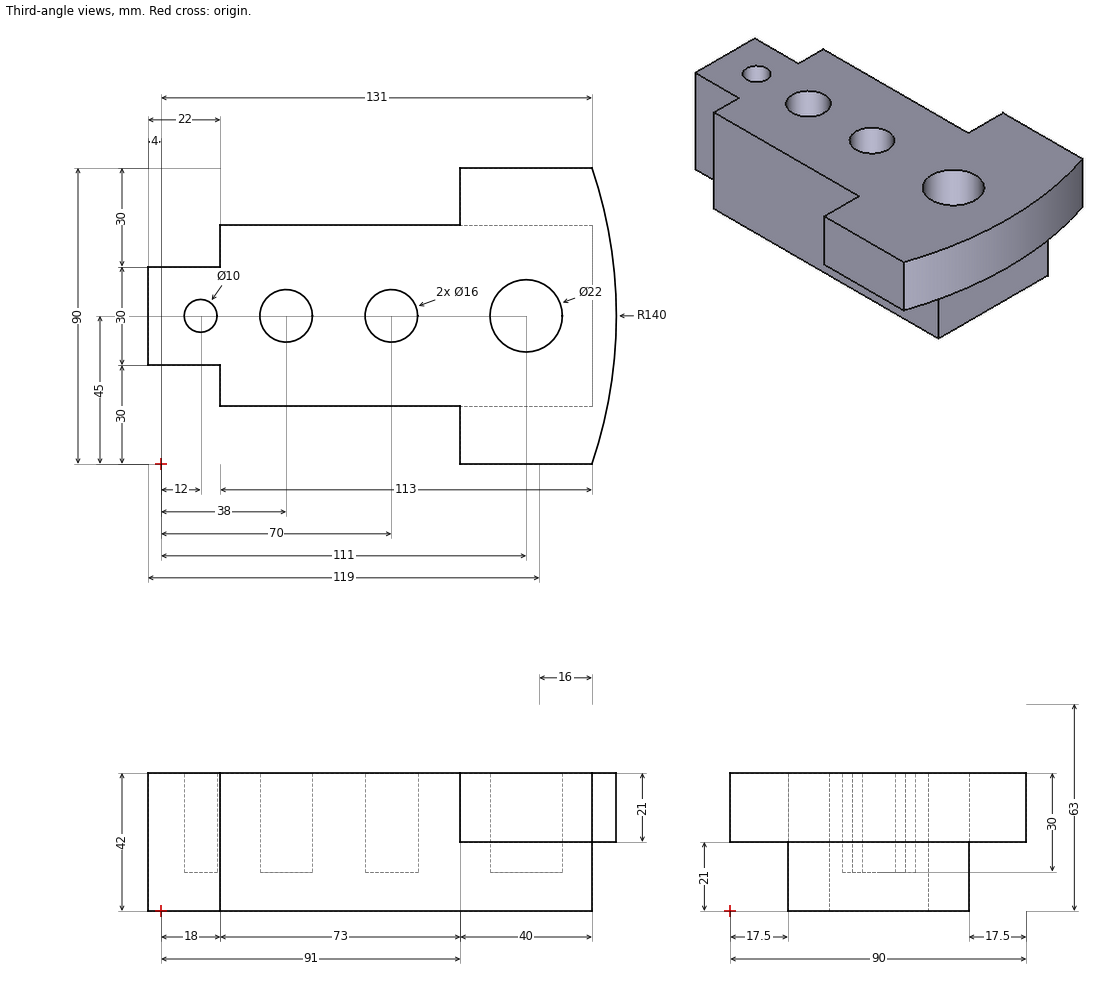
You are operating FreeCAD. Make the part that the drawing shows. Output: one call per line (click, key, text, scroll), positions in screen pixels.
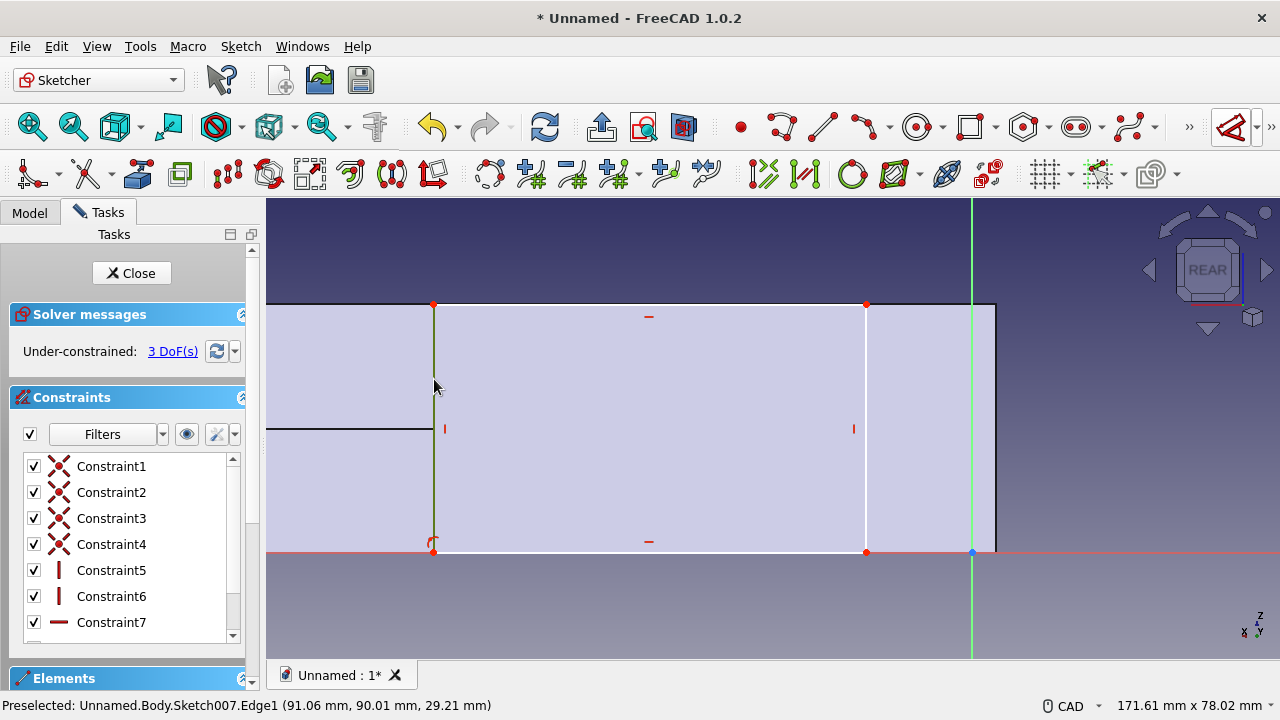
key(i)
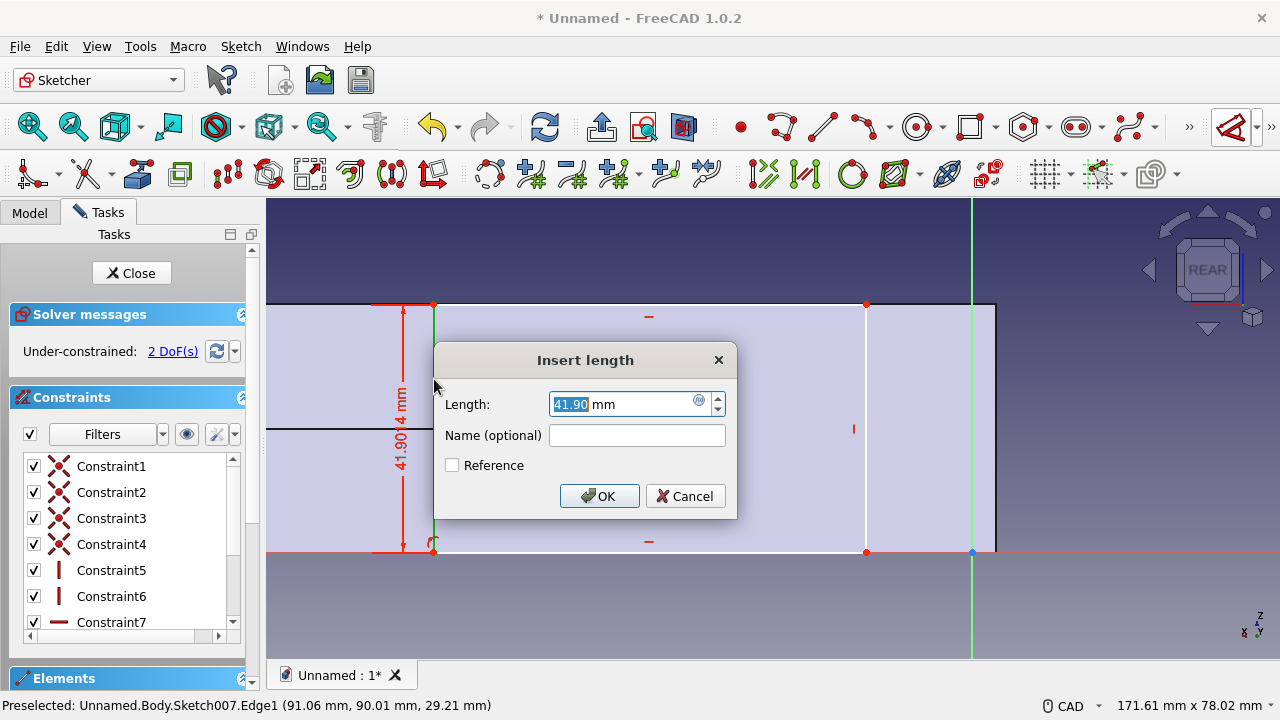
text(42)
key(Return)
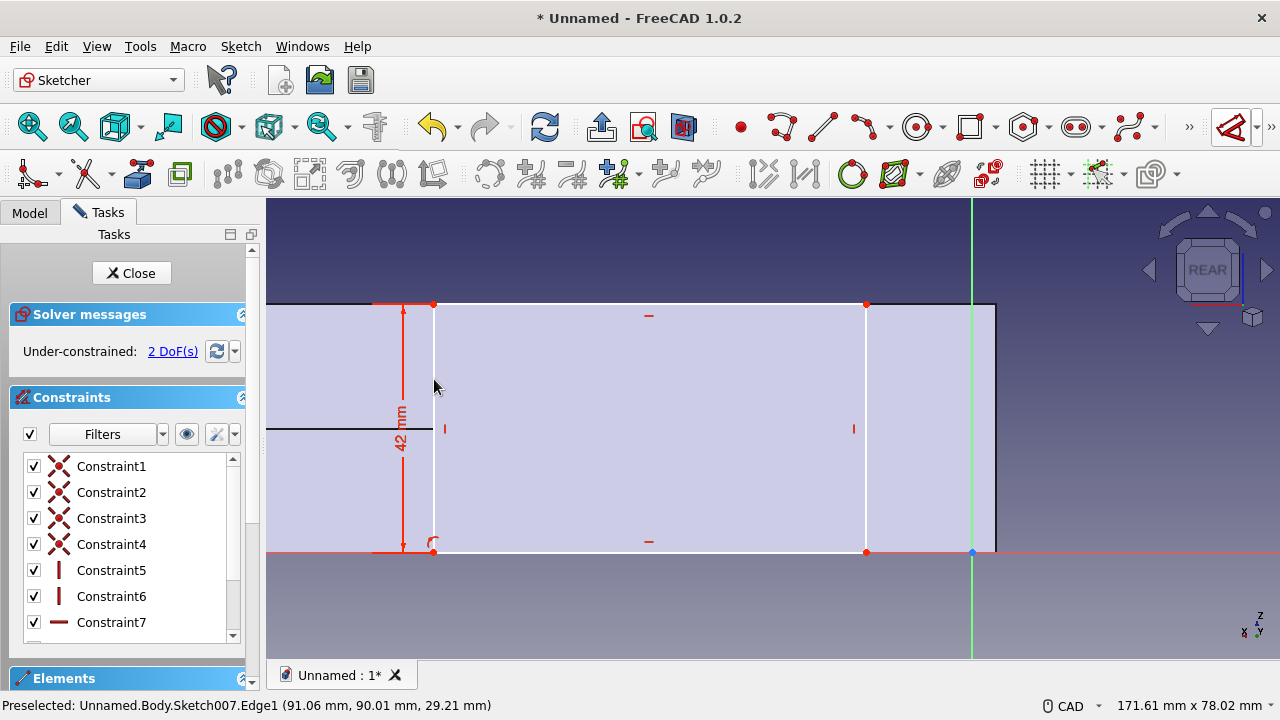
click(564, 553)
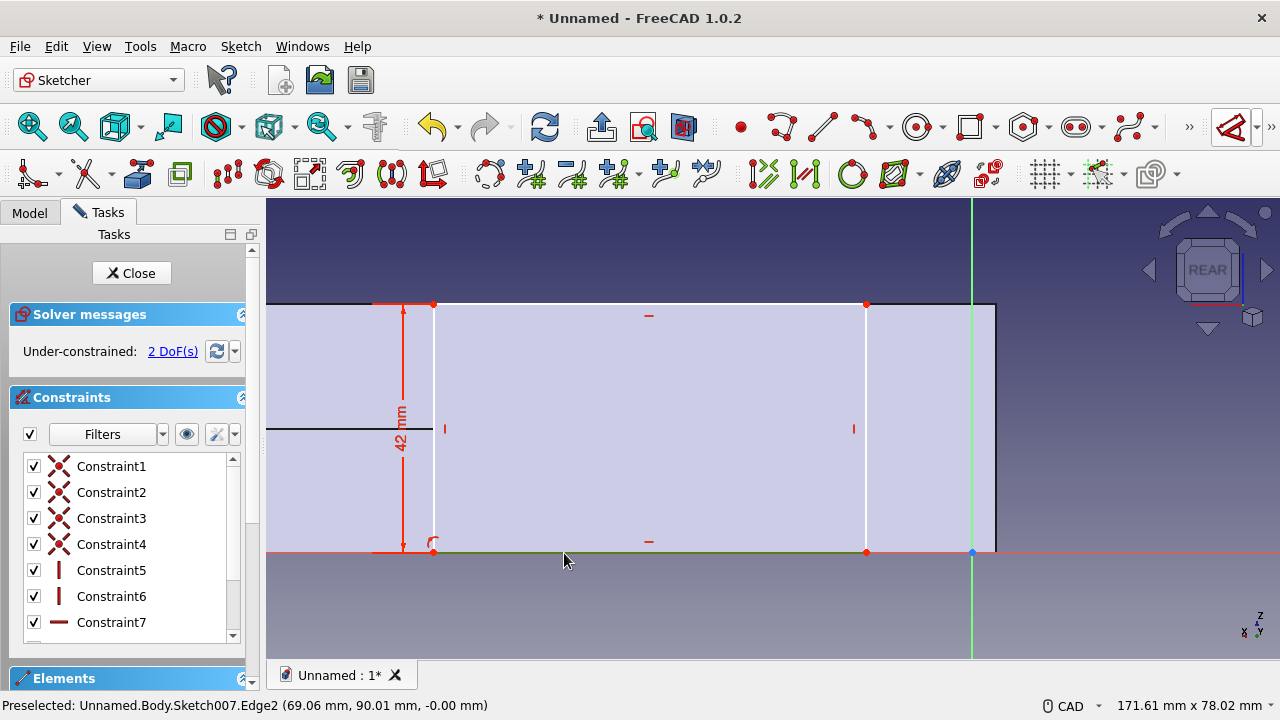
click(1256, 128)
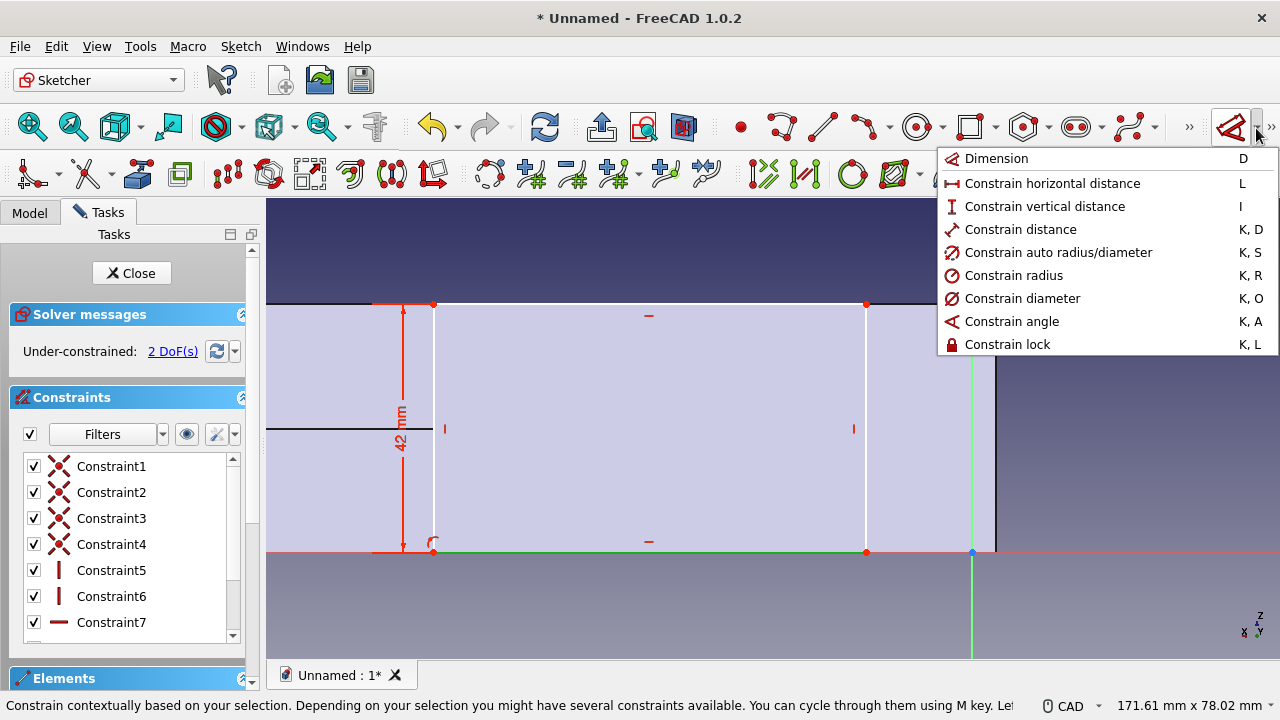
click(1108, 184)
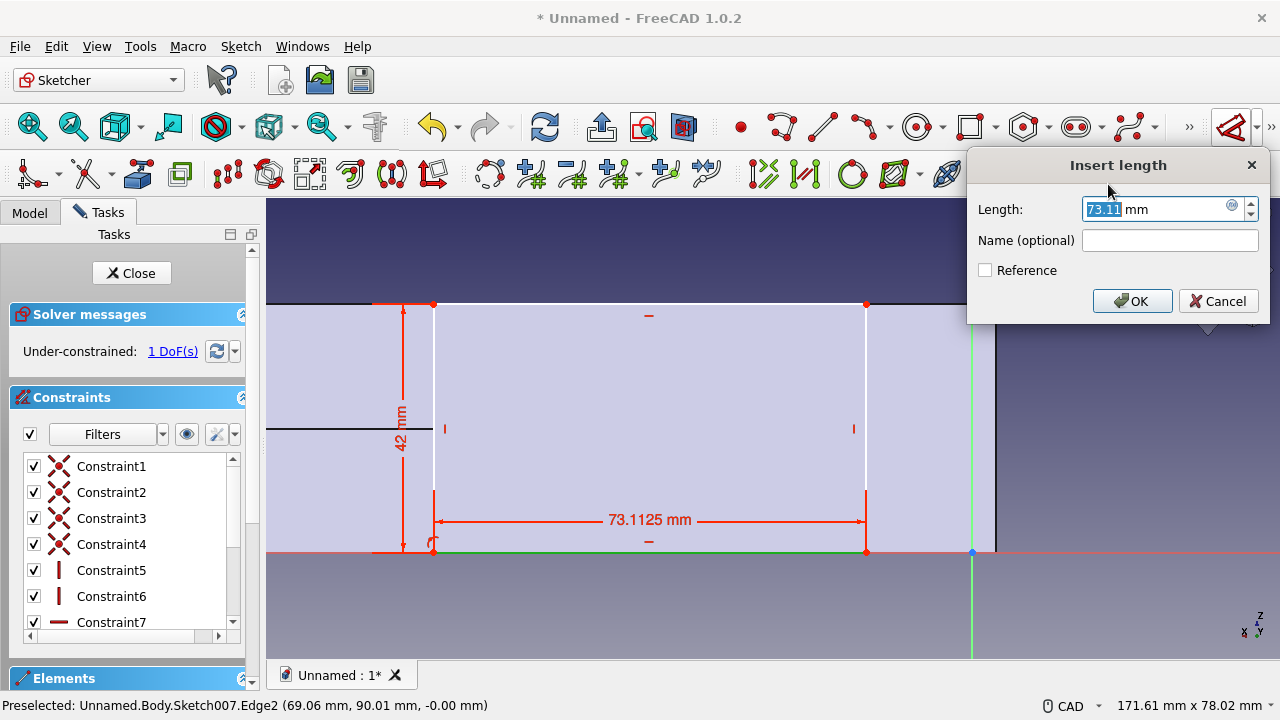
text(73)
key(Return)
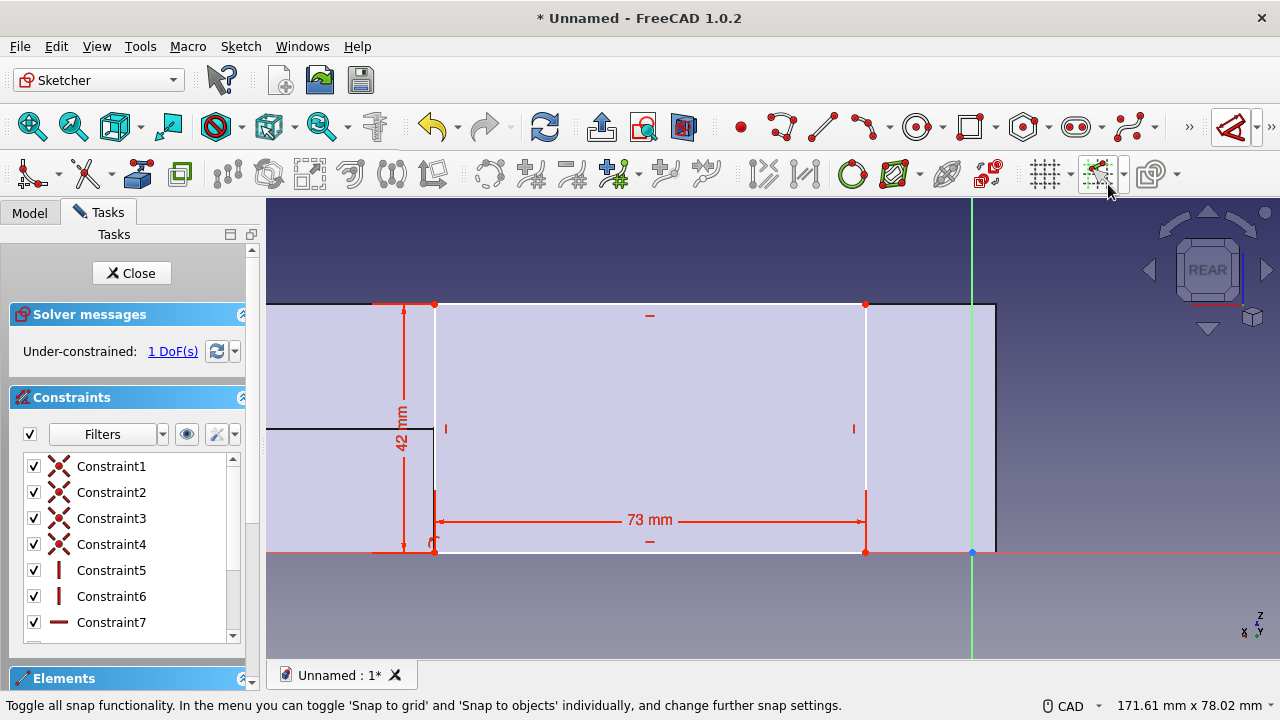
click(435, 304)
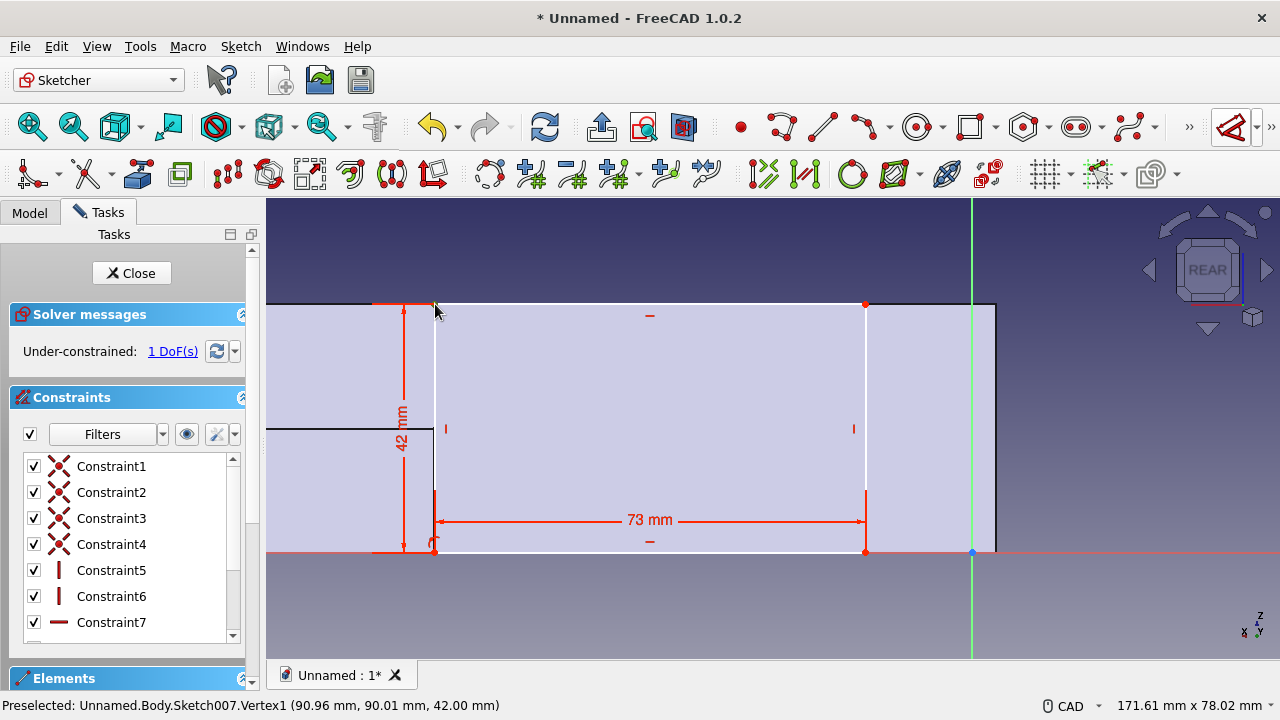
click(1256, 128)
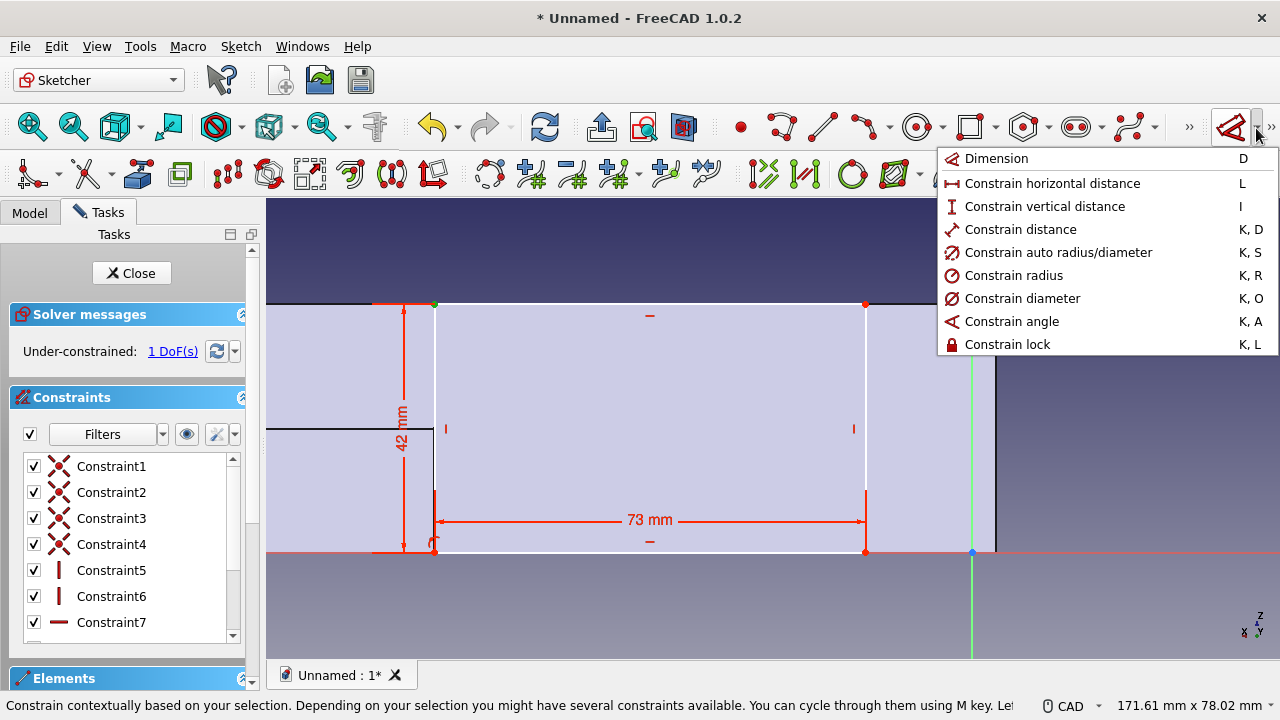
click(1108, 184)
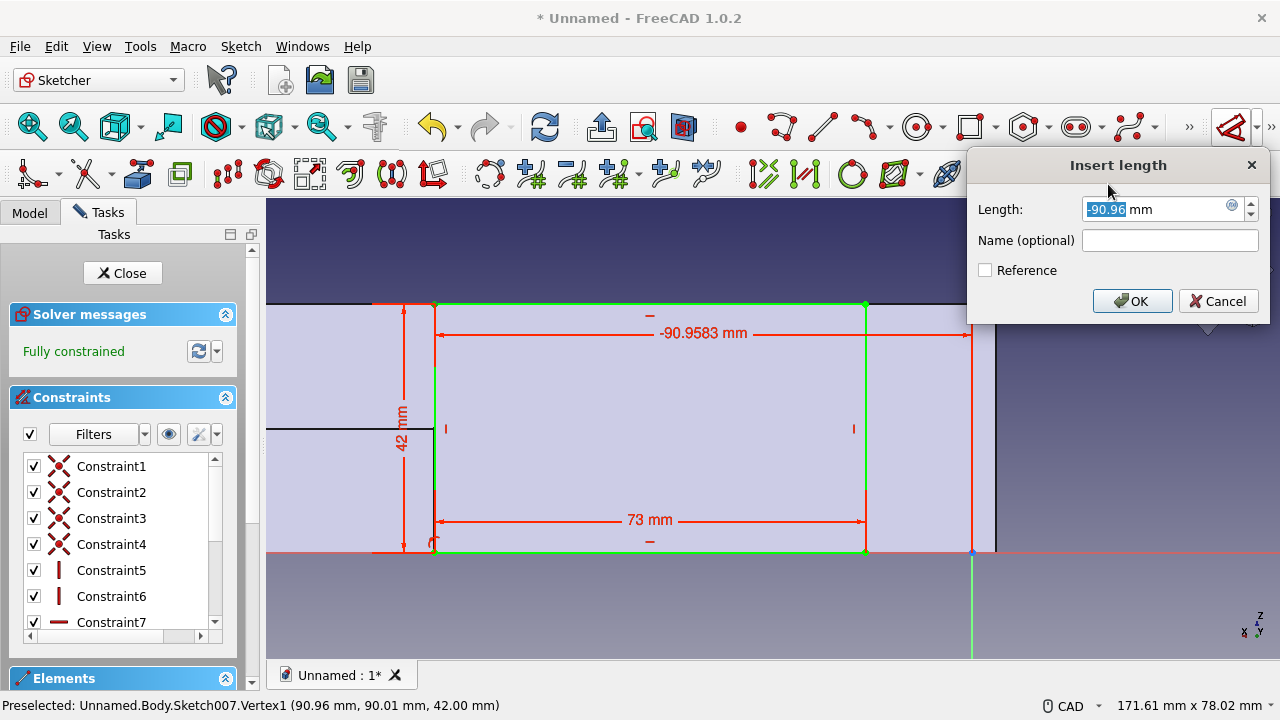
text(-91)
key(Return)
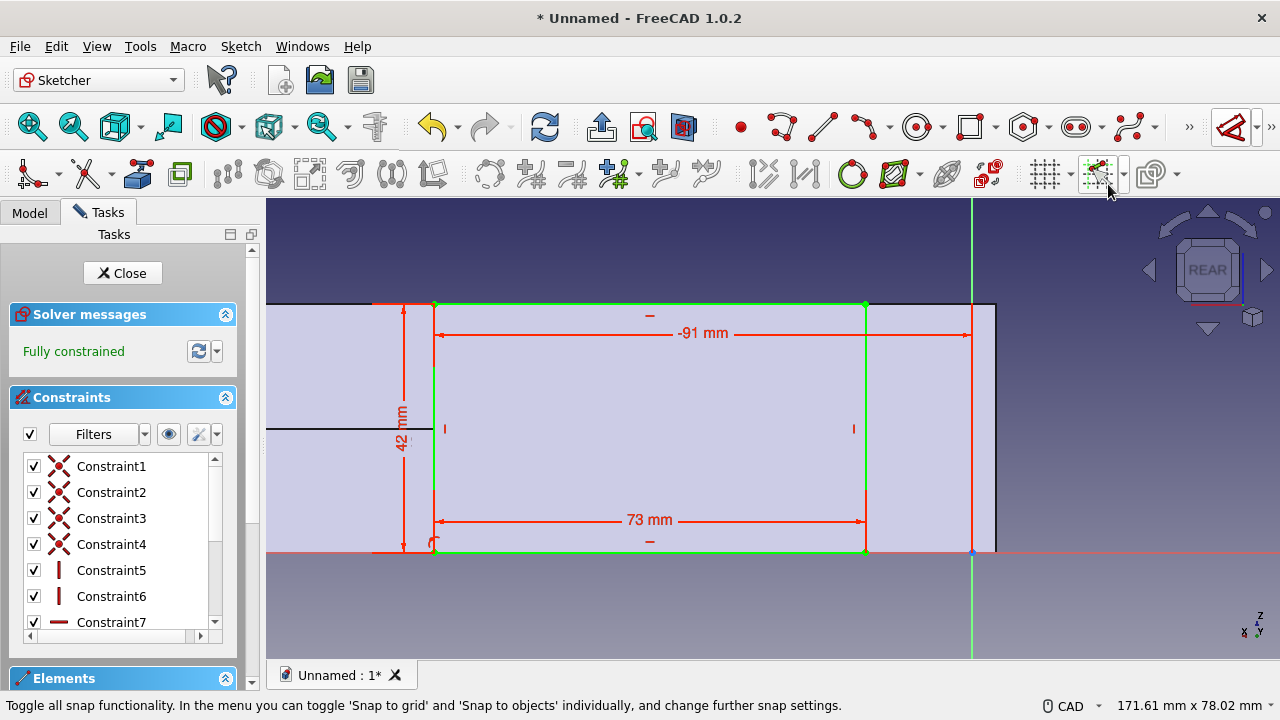
click(123, 273)